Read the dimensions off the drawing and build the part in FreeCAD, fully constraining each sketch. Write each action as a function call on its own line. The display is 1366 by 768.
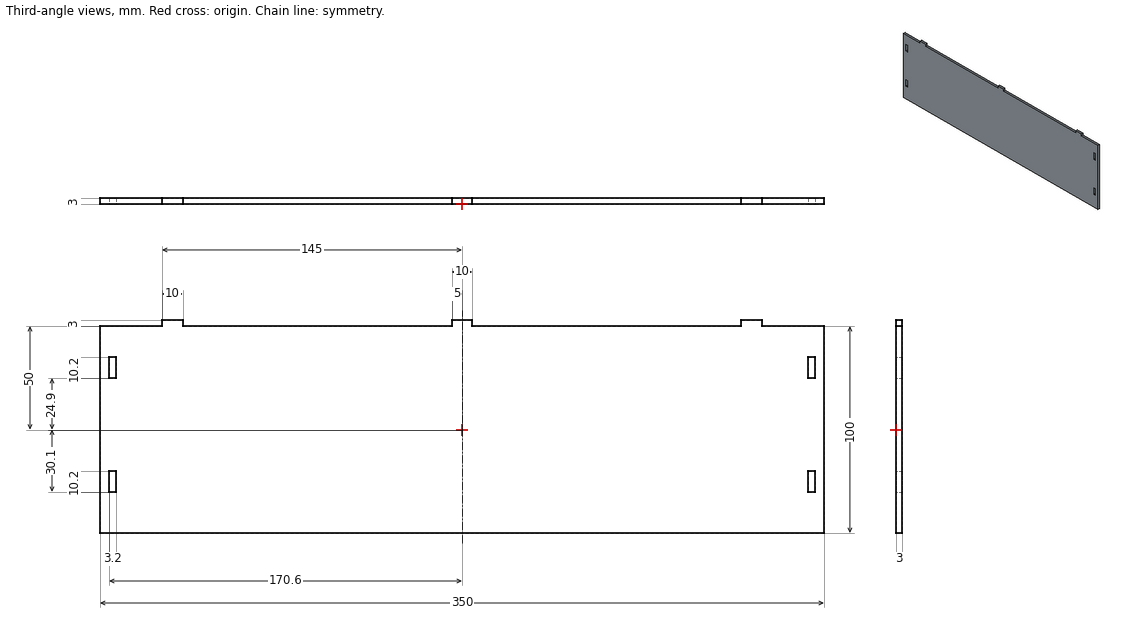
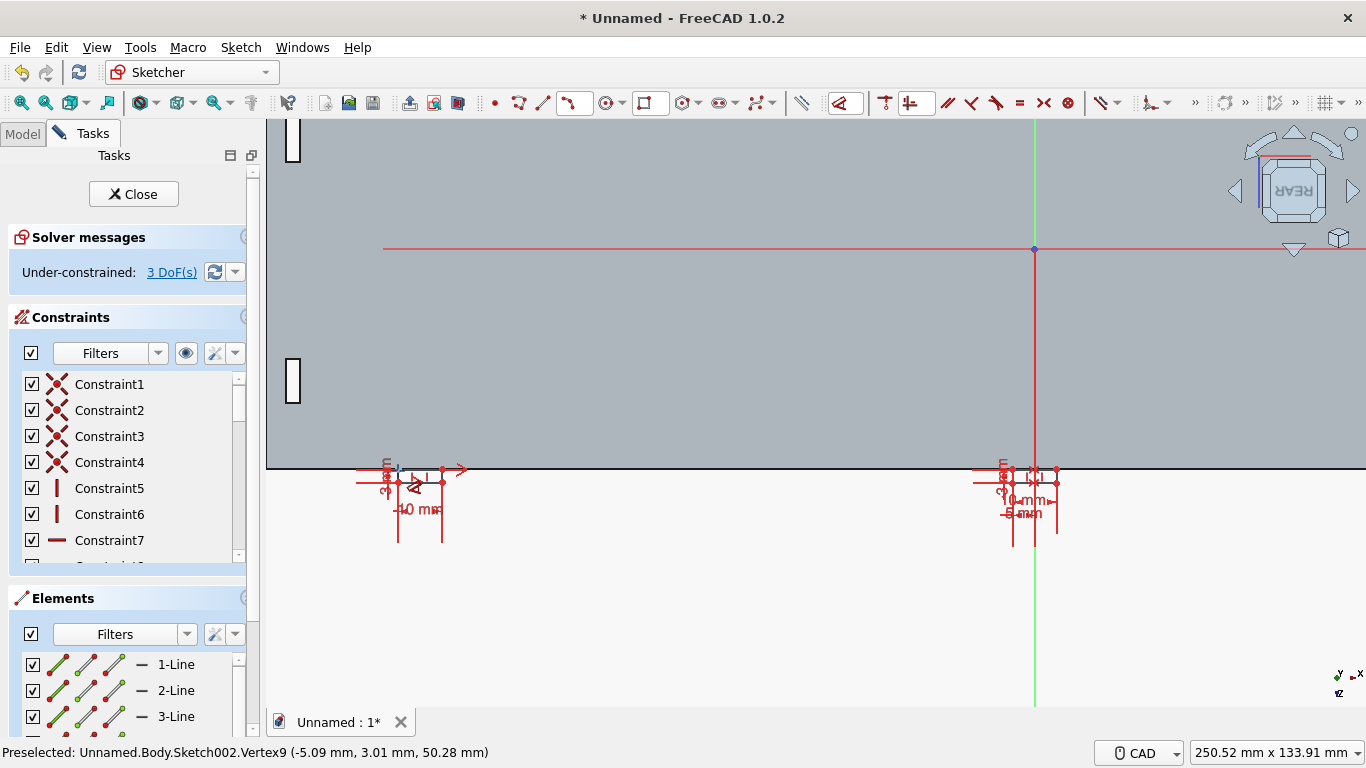
click(398, 470)
click(364, 359)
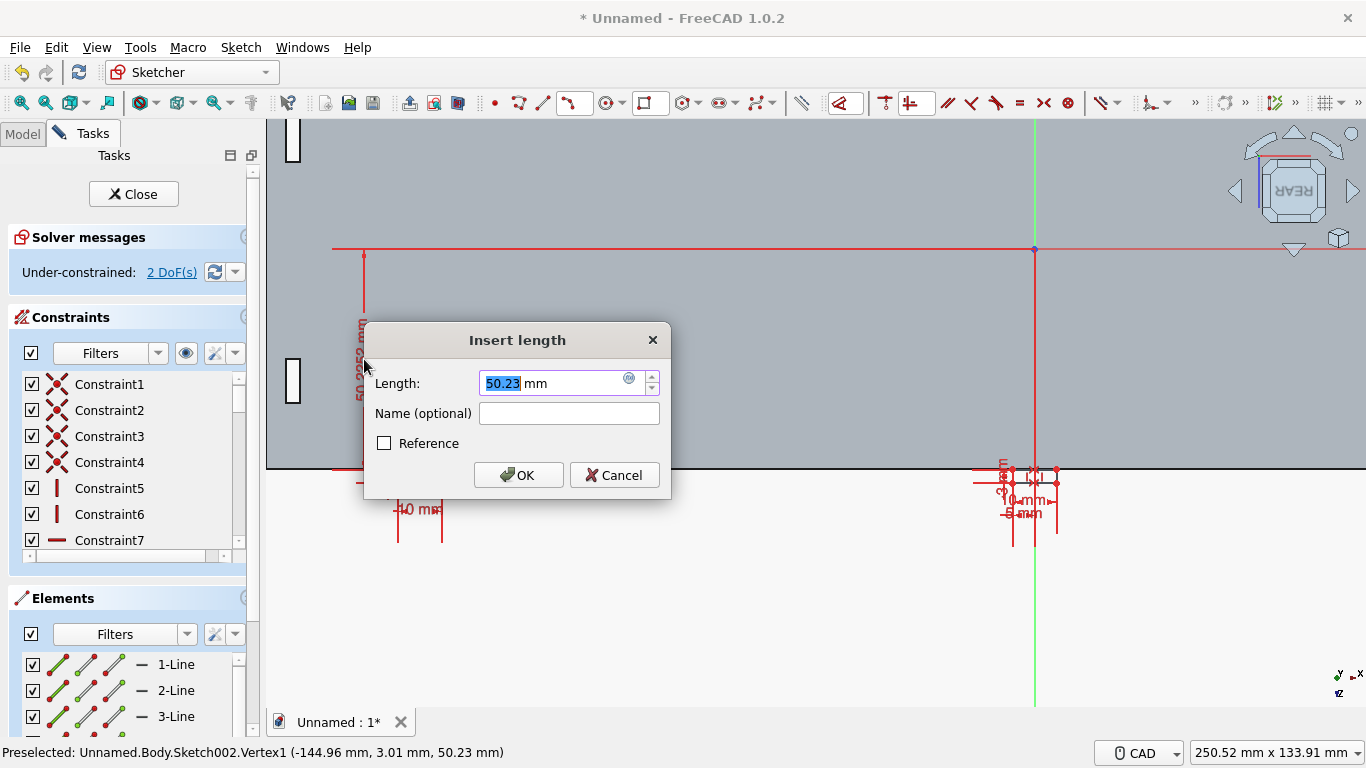
text(50)
key(Return)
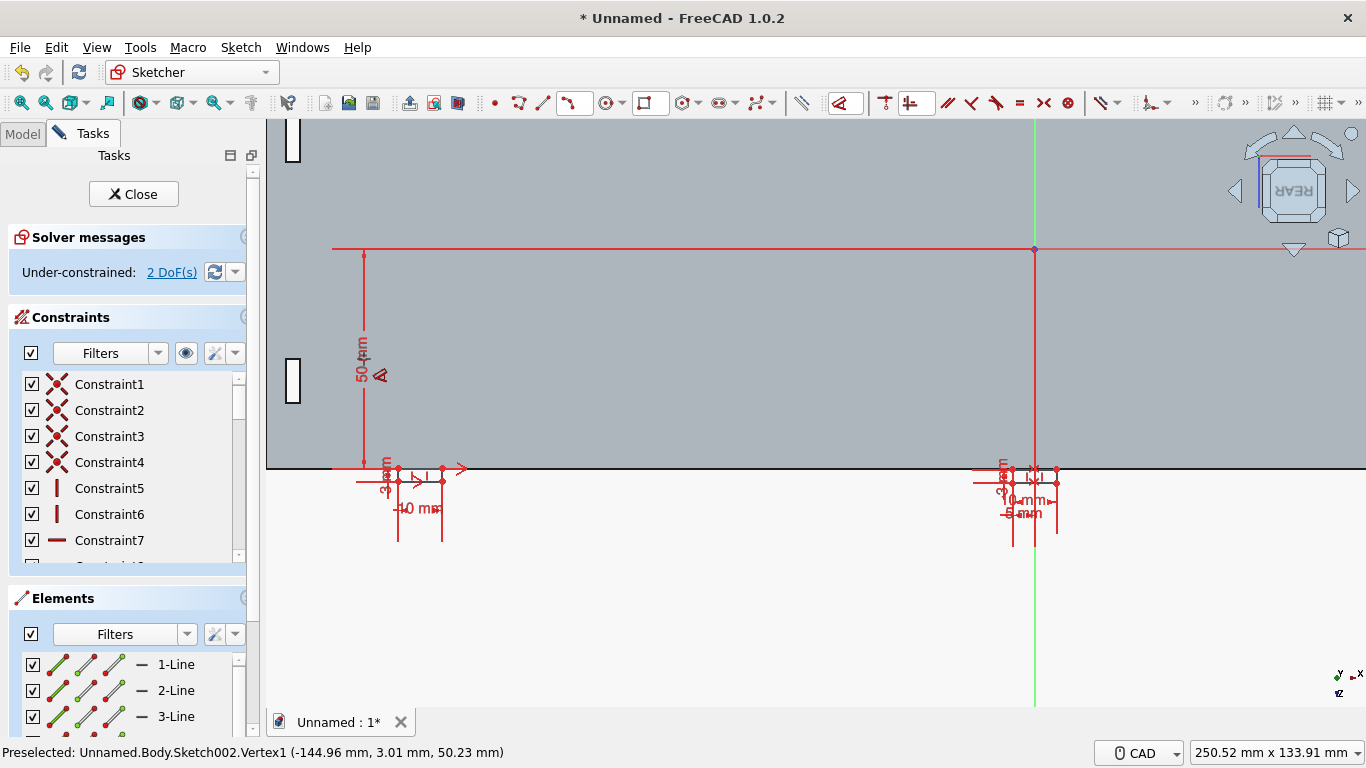
click(1013, 470)
click(979, 360)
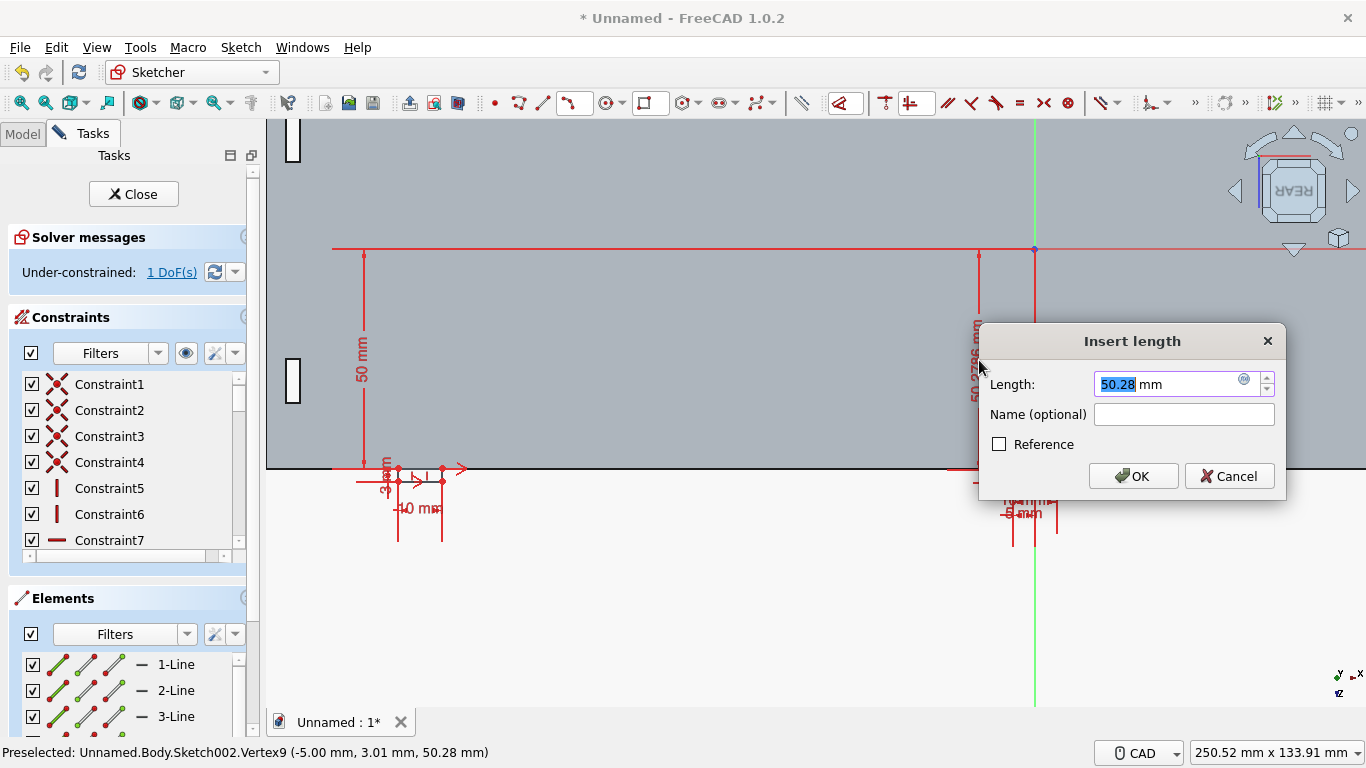
text(50)
key(Return)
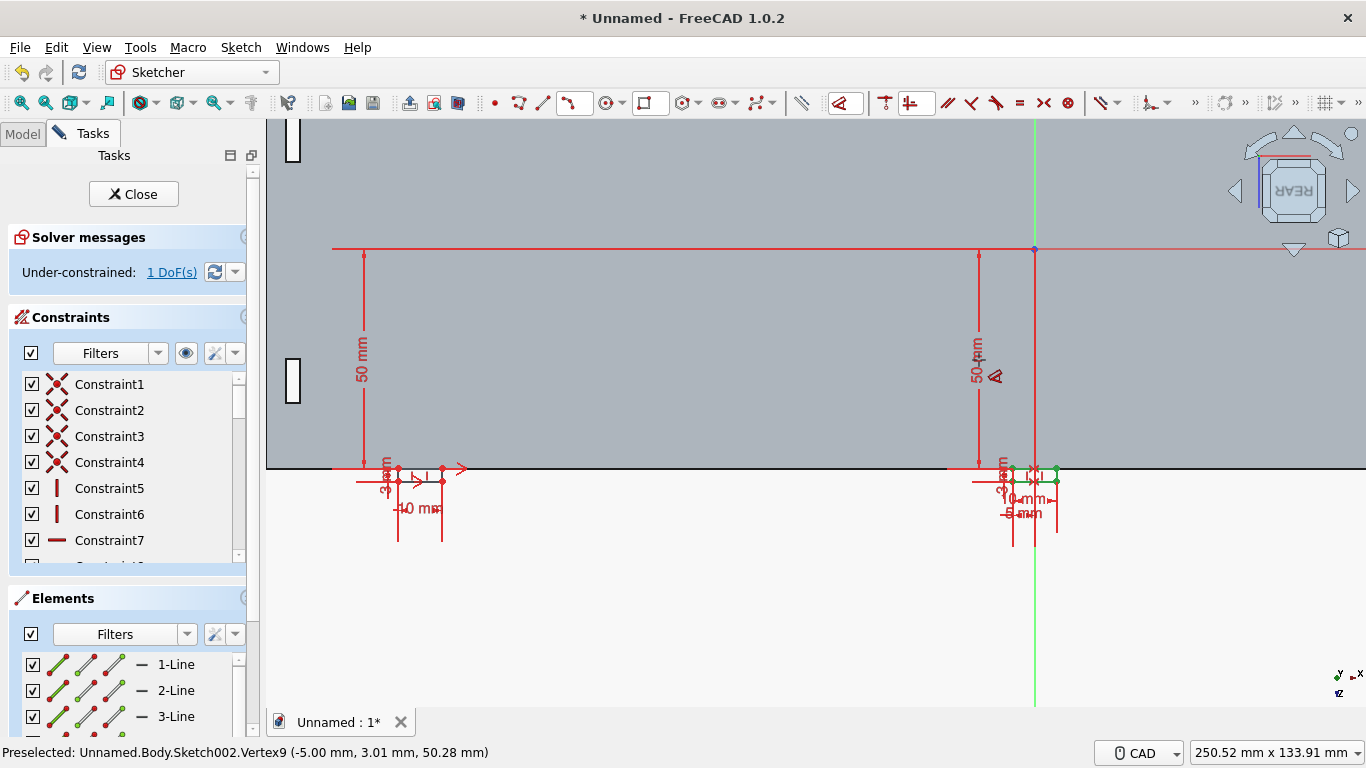
click(398, 469)
click(717, 215)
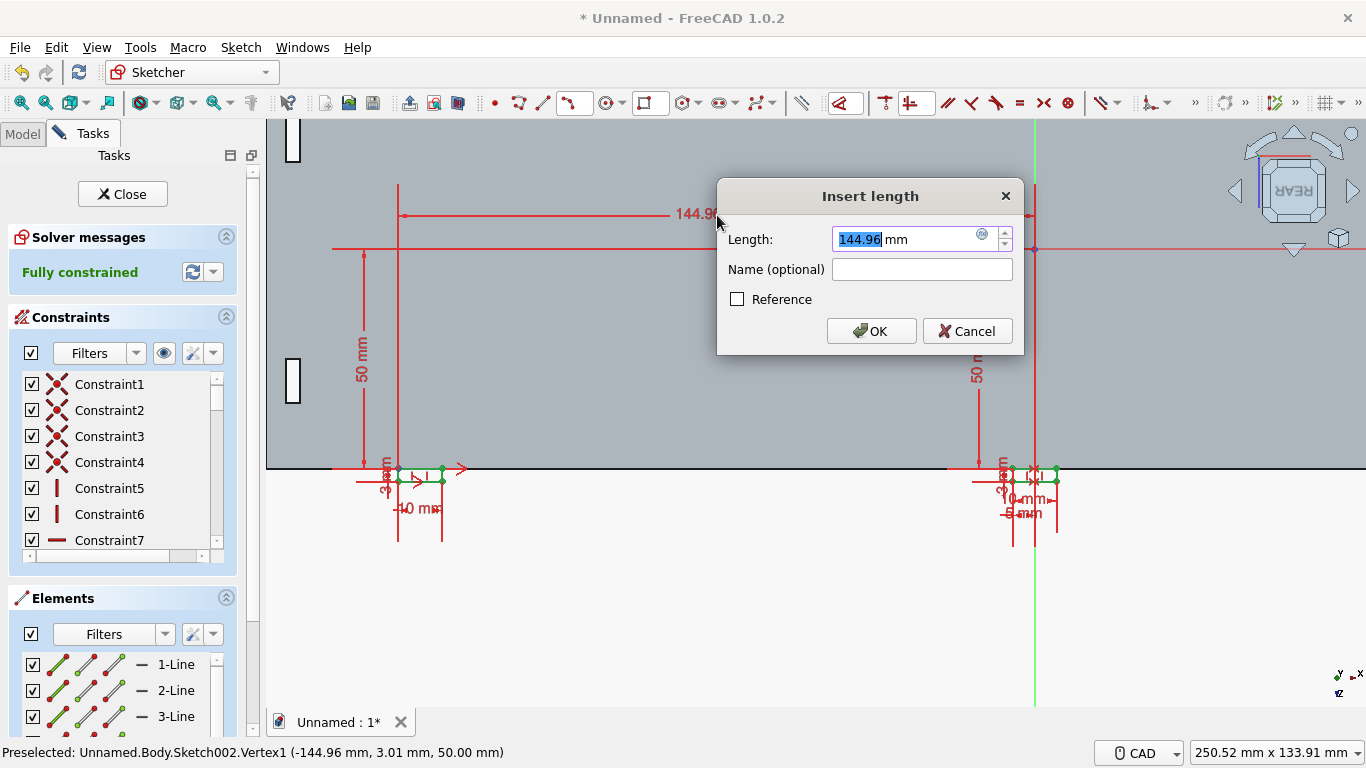
text(145)
key(Return)
key(Escape)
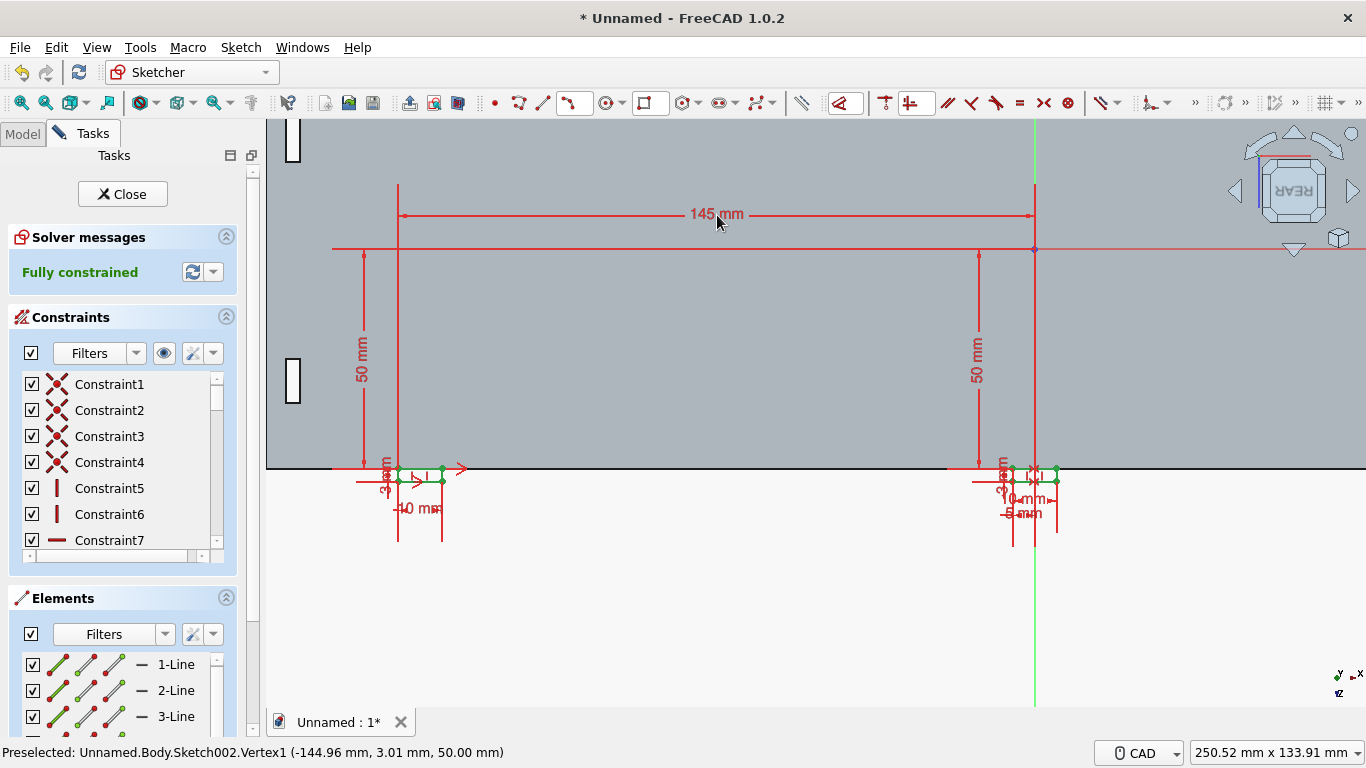
click(123, 194)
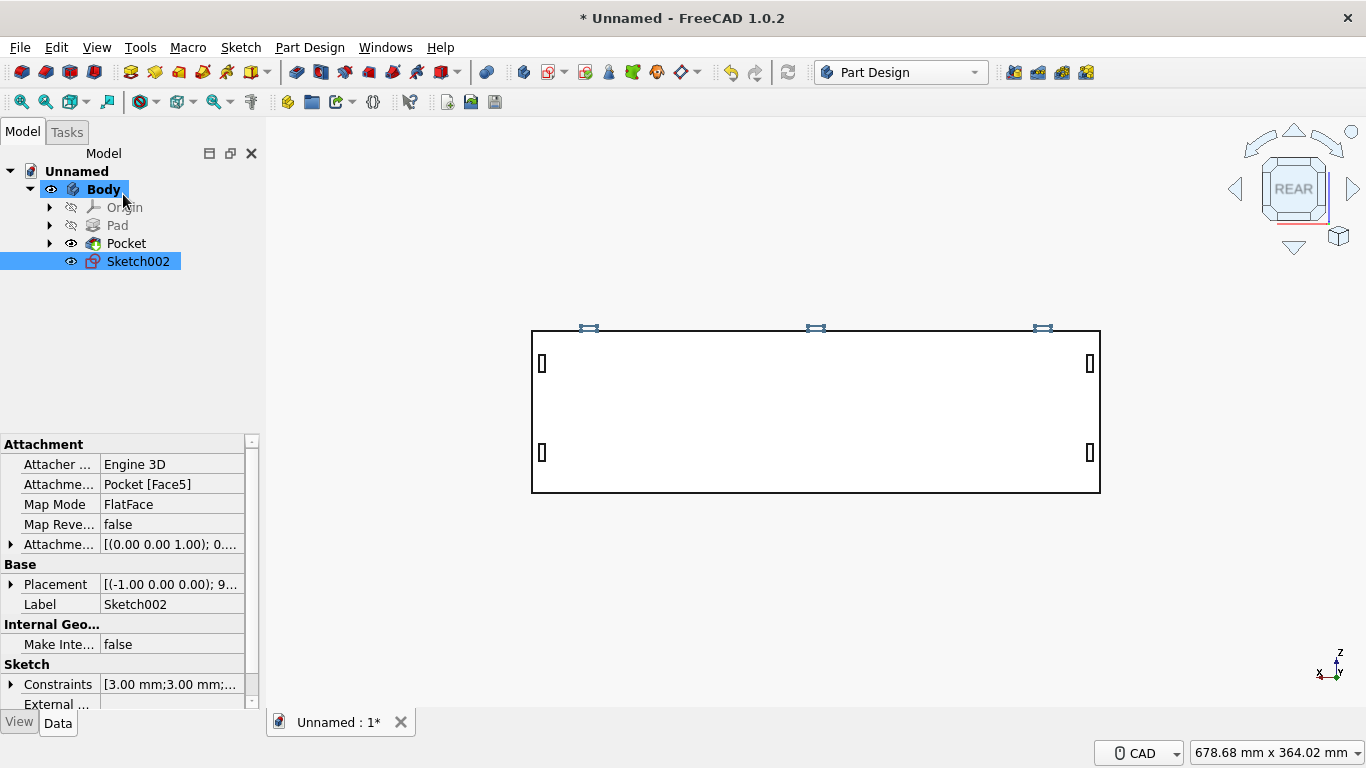
click(132, 72)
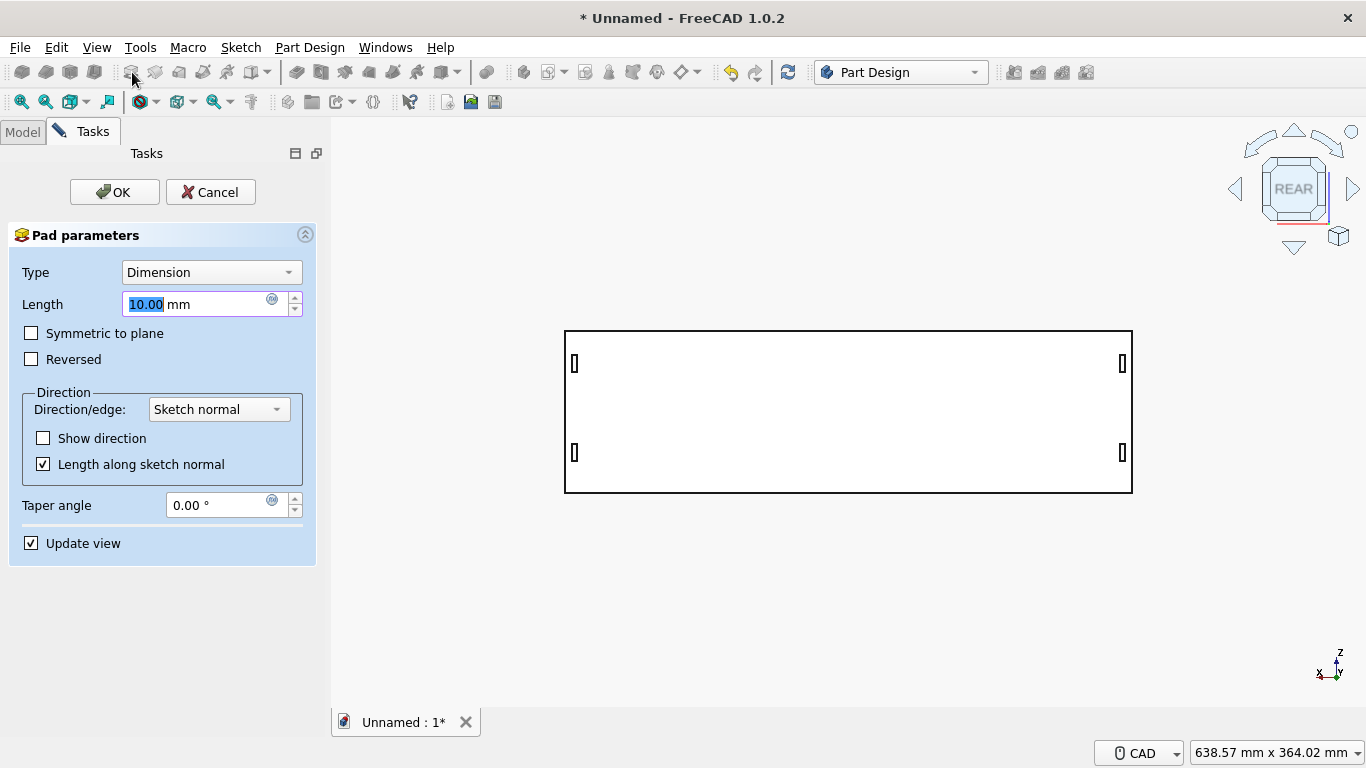
text(3)
key(Tab)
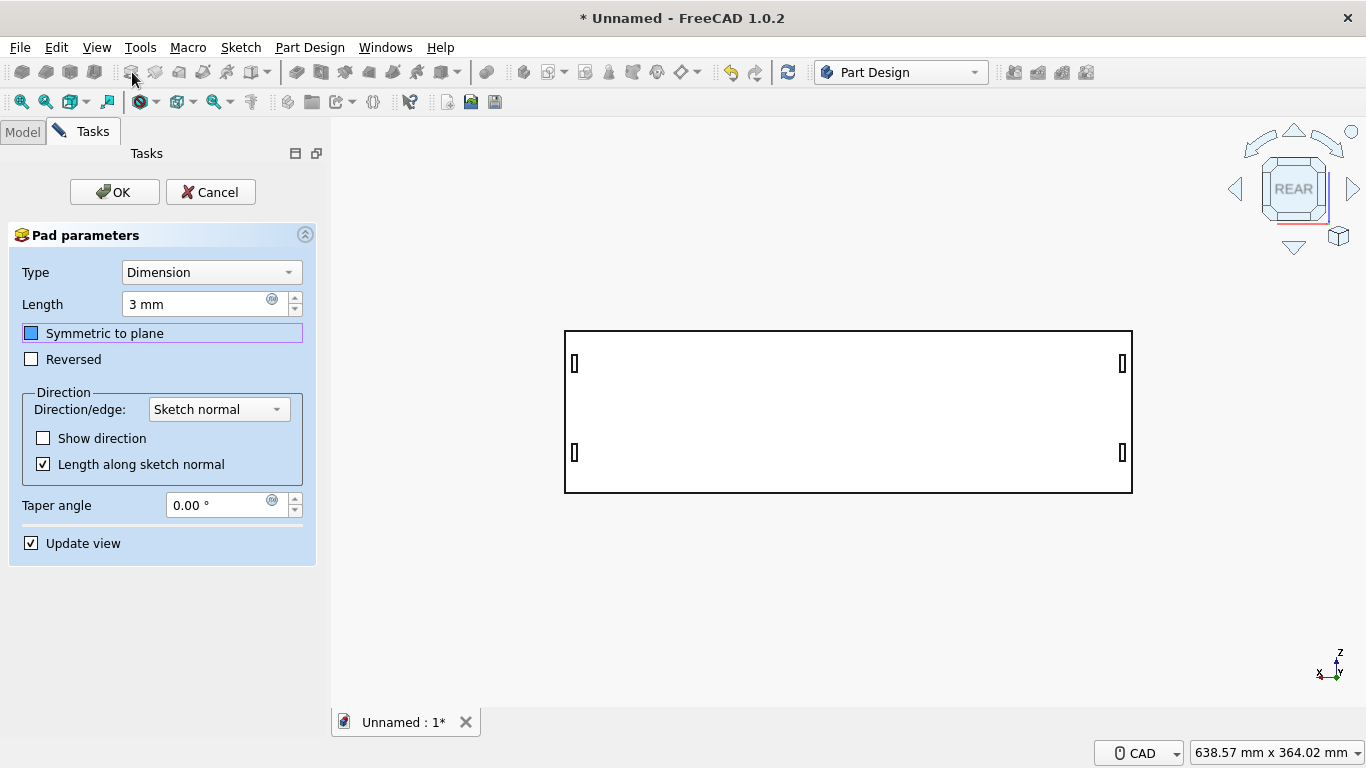
click(30, 359)